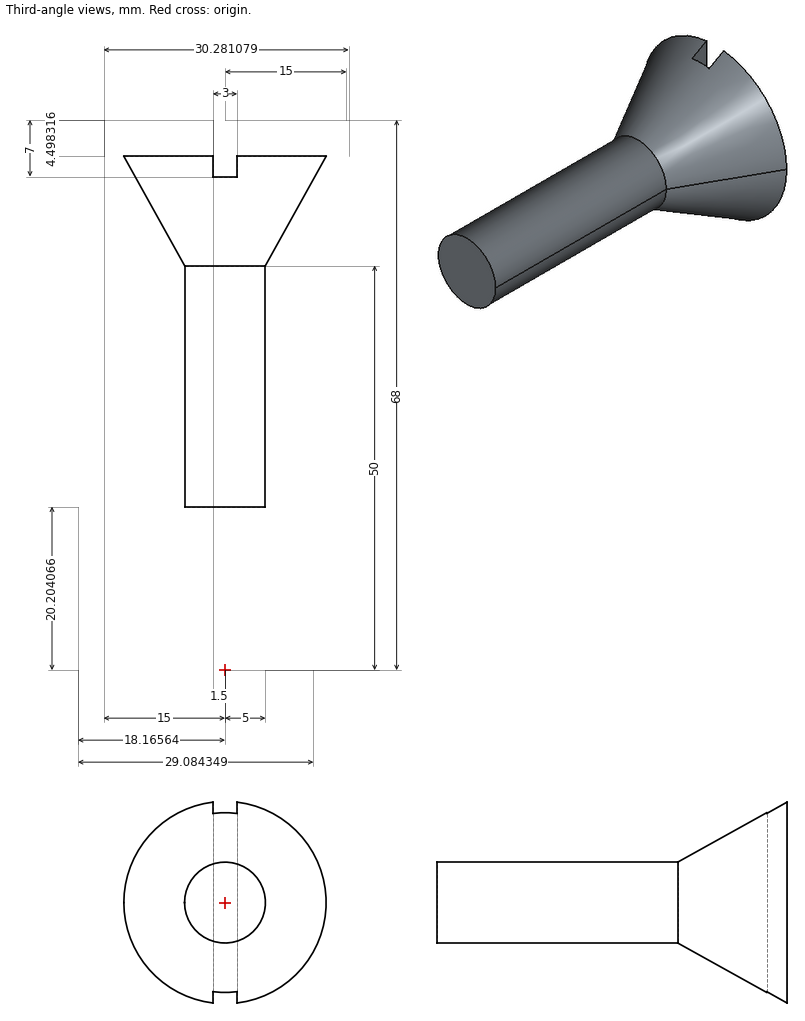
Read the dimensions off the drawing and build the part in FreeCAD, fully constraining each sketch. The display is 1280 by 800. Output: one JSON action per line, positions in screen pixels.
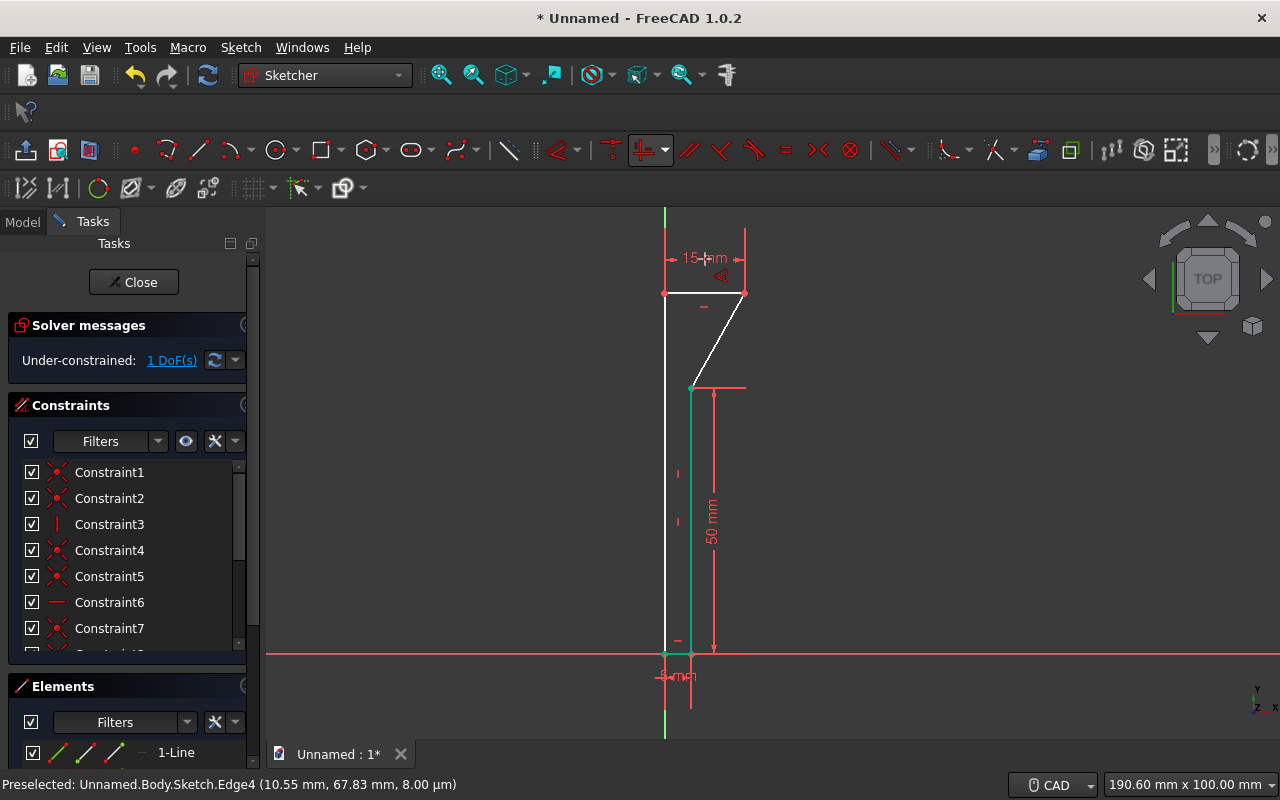
{"action": "left_click", "coordinate": [665, 402]}
{"action": "left_click", "coordinate": [631, 474]}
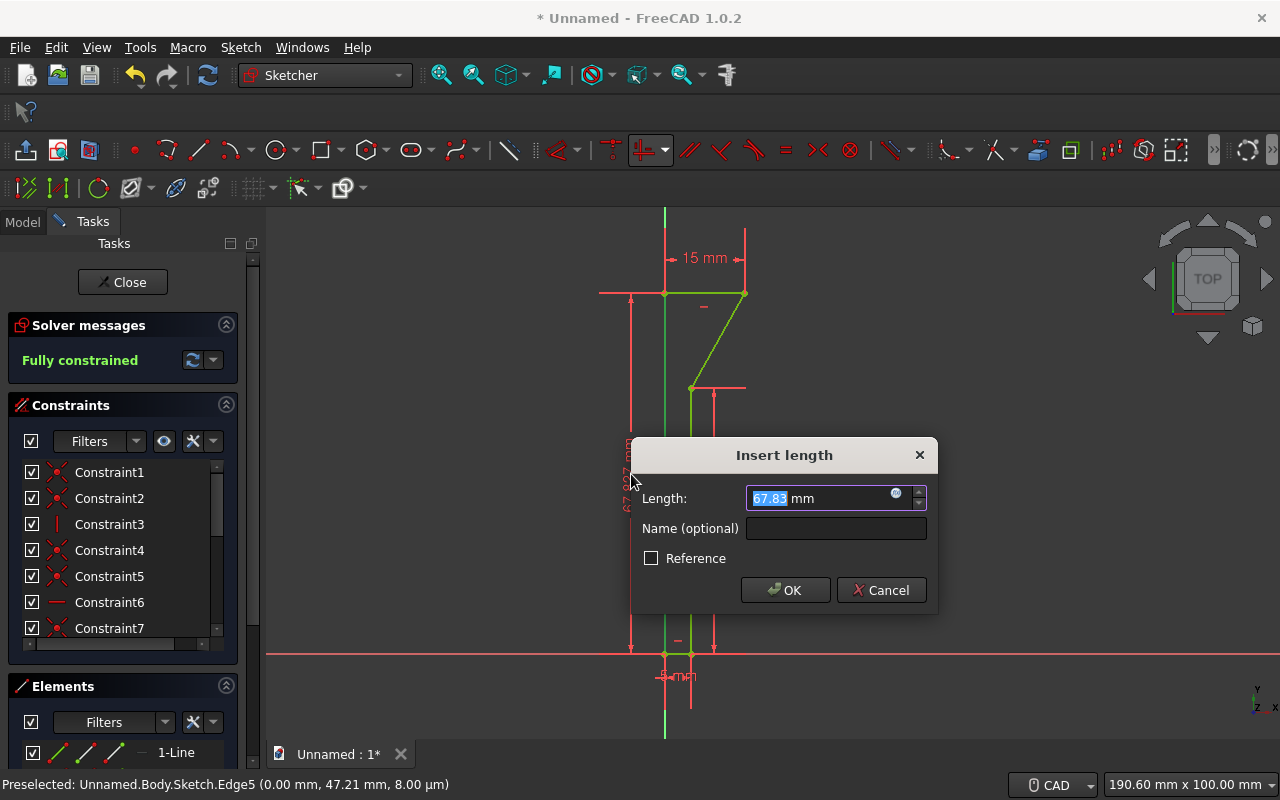
{"action": "type", "text": "68"}
{"action": "key", "text": "Return"}
{"action": "key", "text": "Escape"}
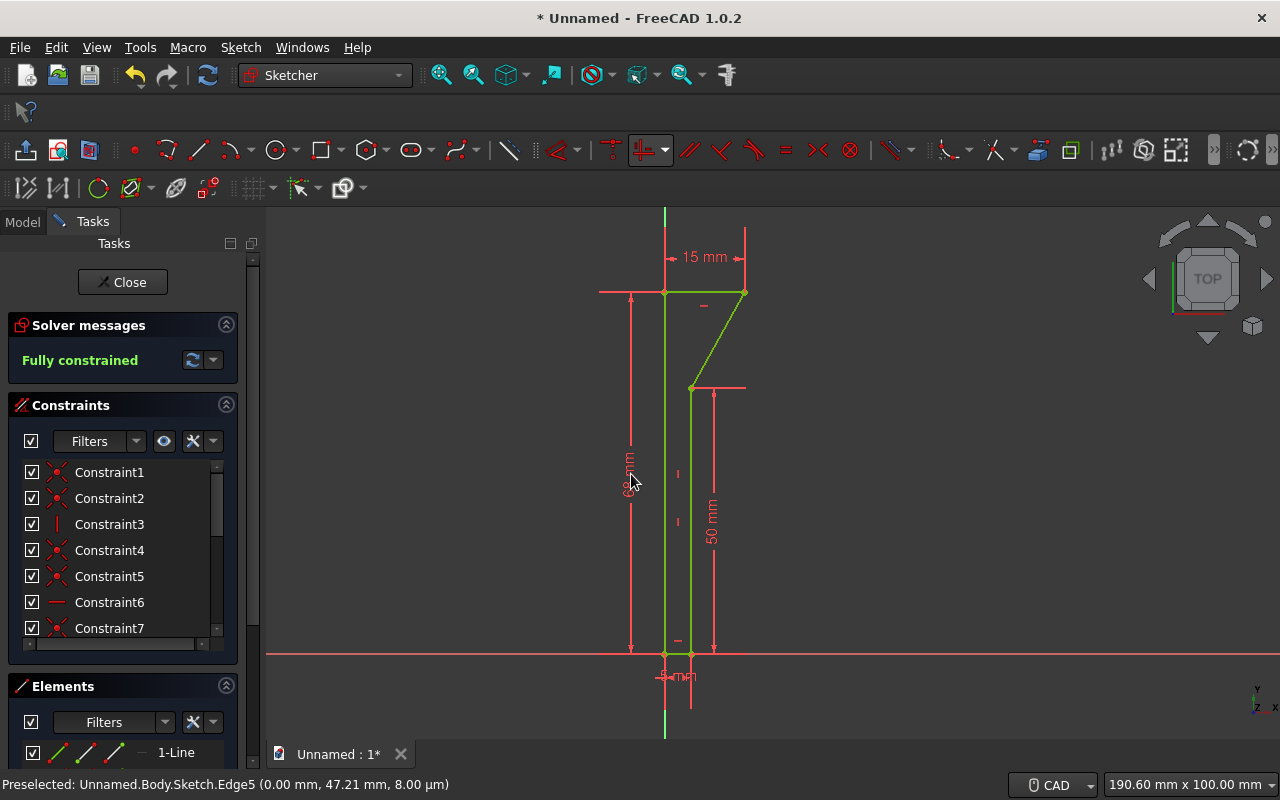
{"action": "left_click", "coordinate": [123, 282]}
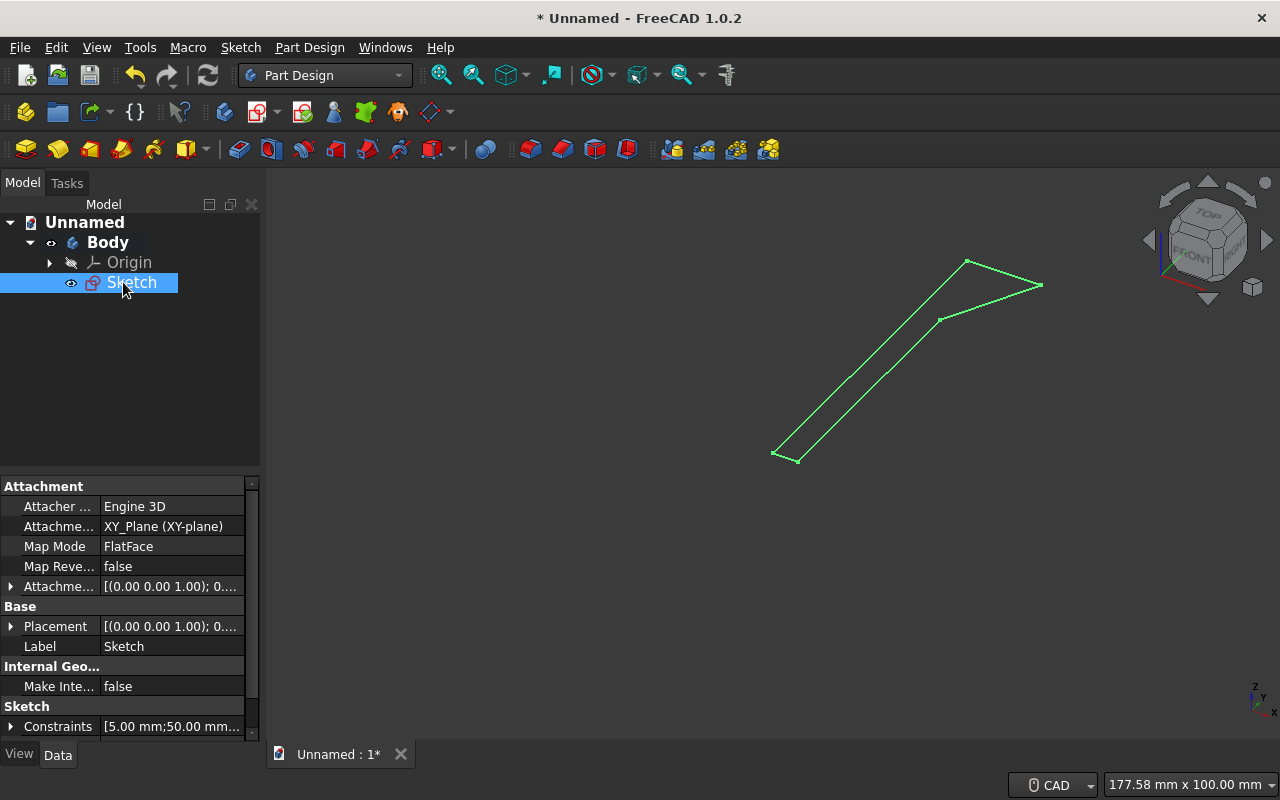
{"action": "left_click", "coordinate": [58, 150]}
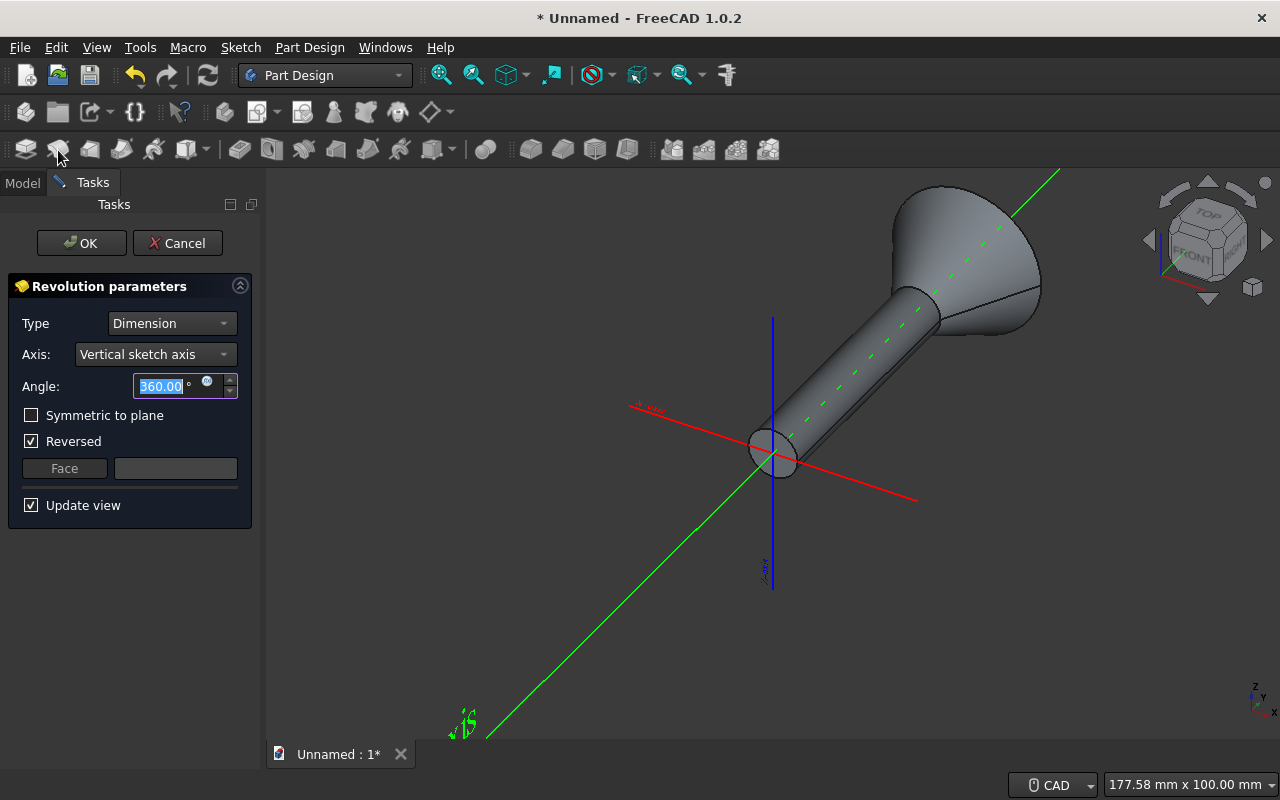
{"action": "left_click", "coordinate": [82, 243]}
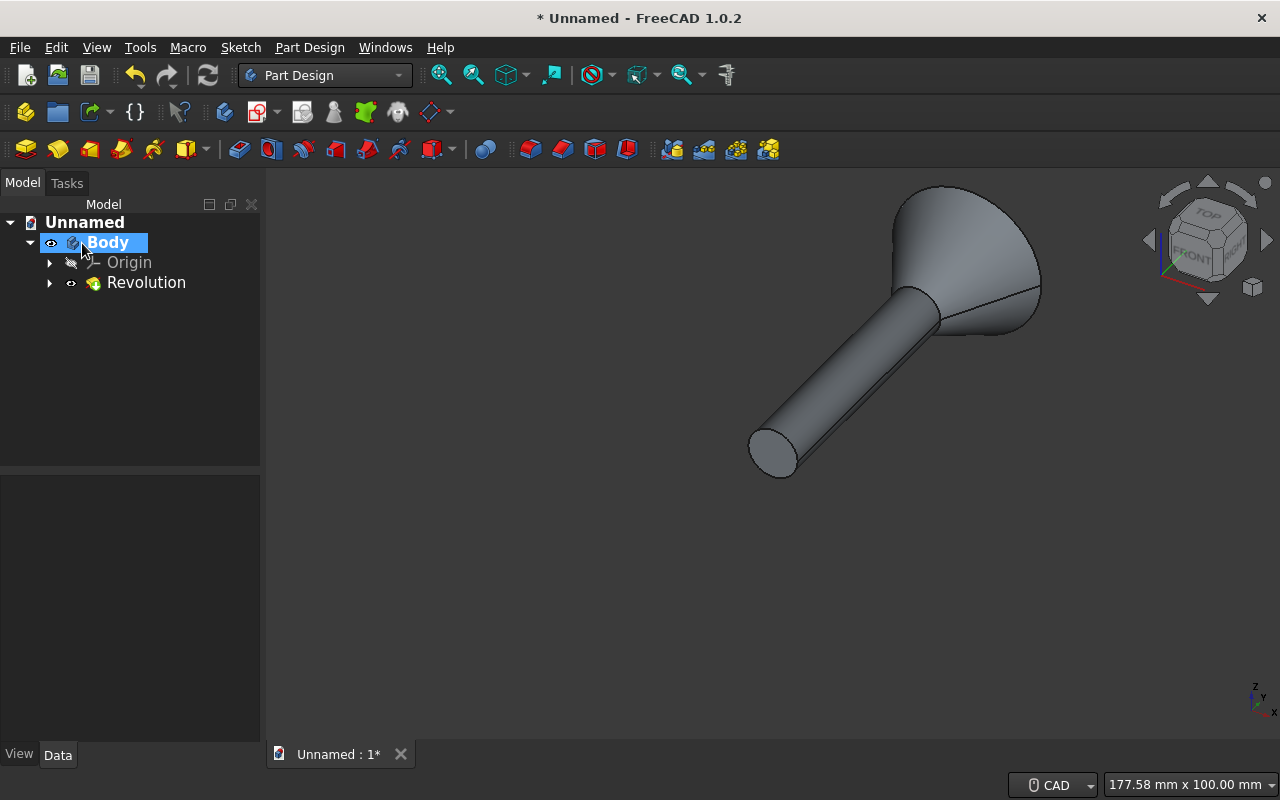
{"action": "left_click", "coordinate": [442, 76]}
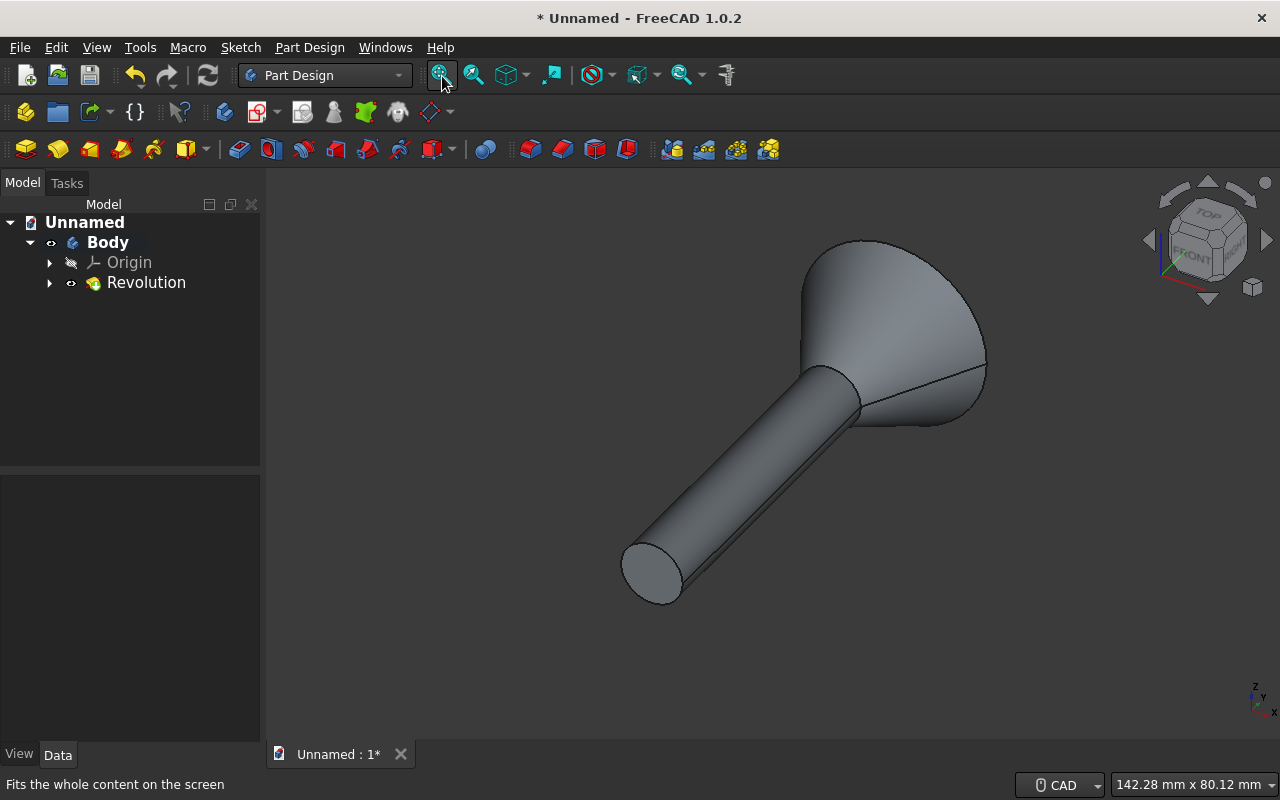
{"action": "left_click", "coordinate": [258, 112]}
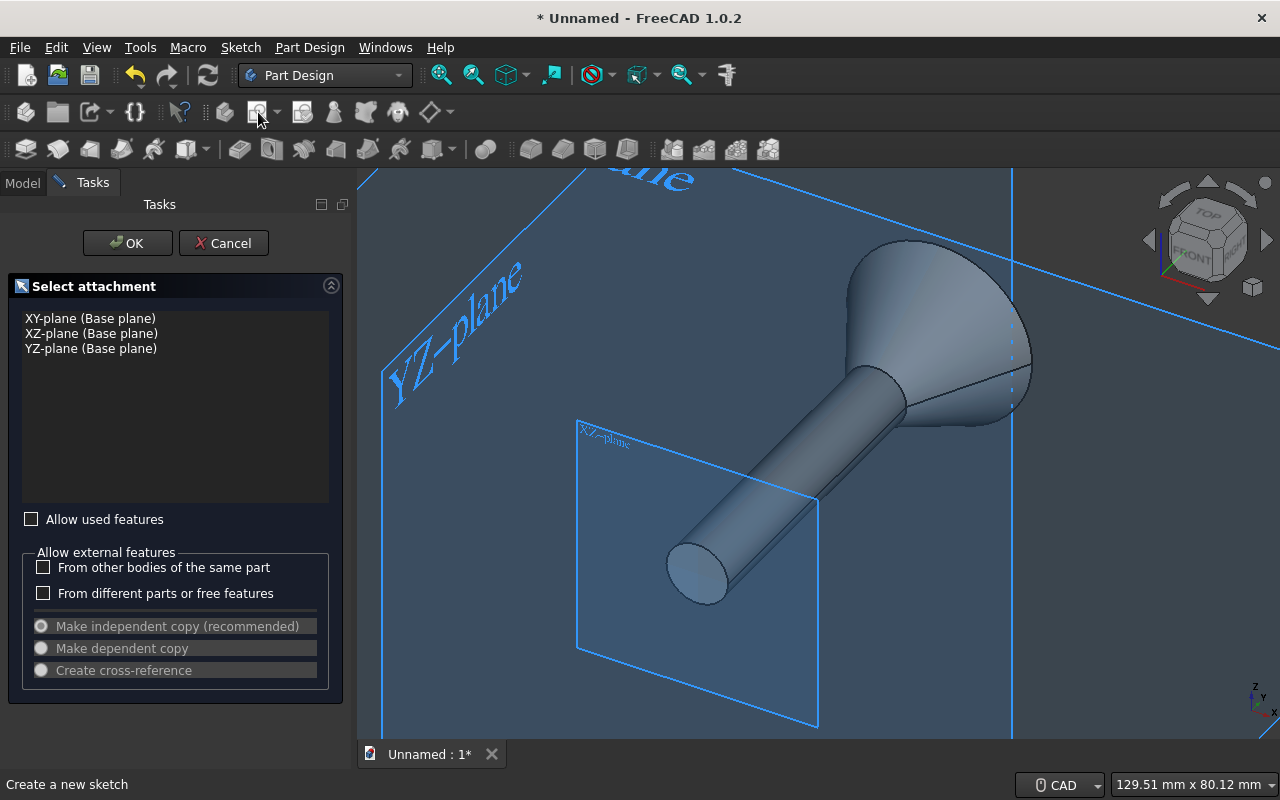
{"action": "left_click", "coordinate": [82, 318]}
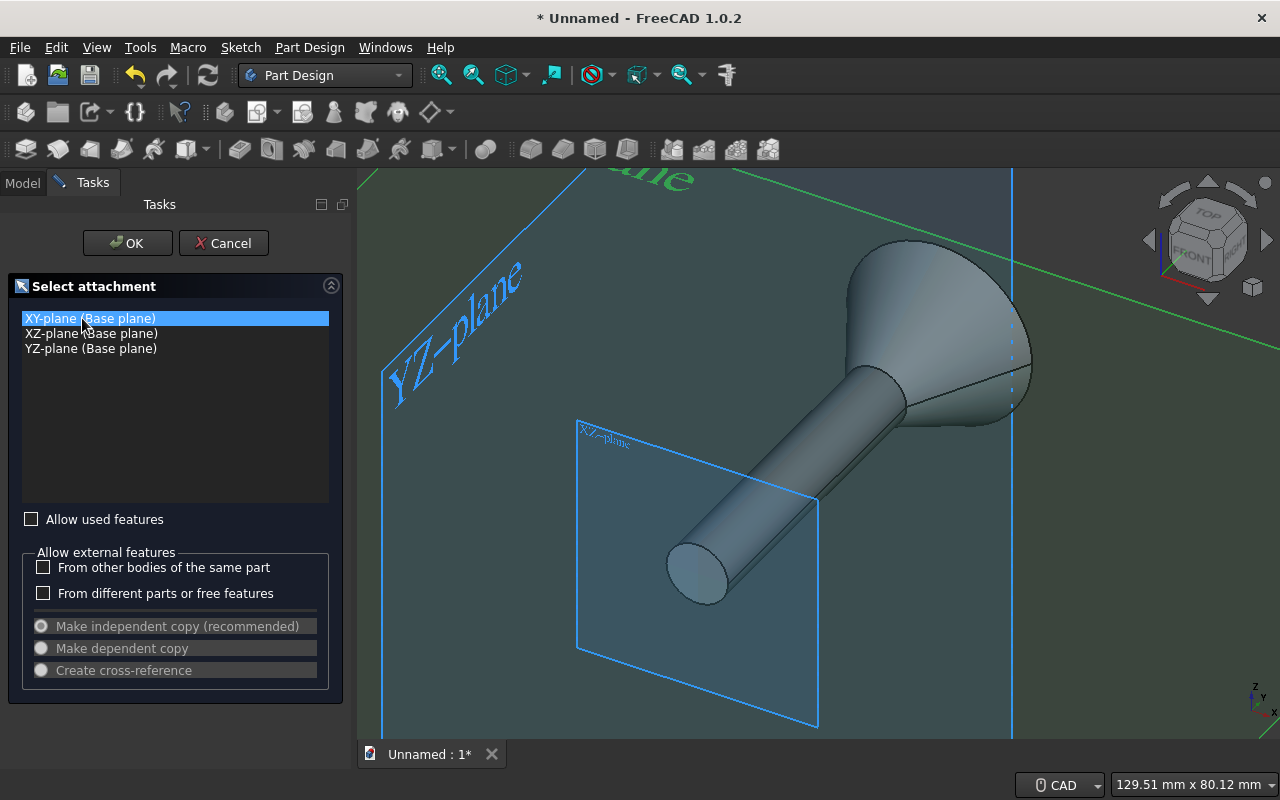
{"action": "left_click", "coordinate": [128, 243]}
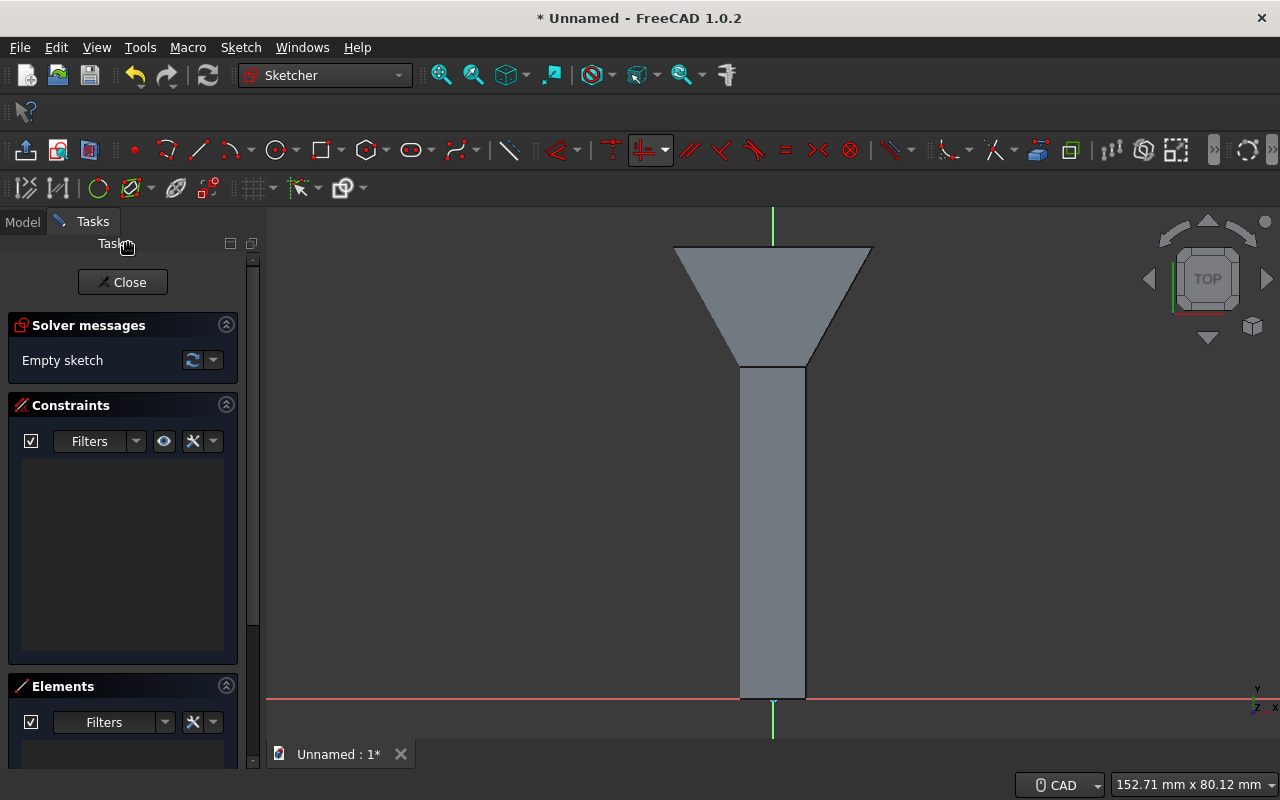
{"action": "left_click", "coordinate": [90, 150]}